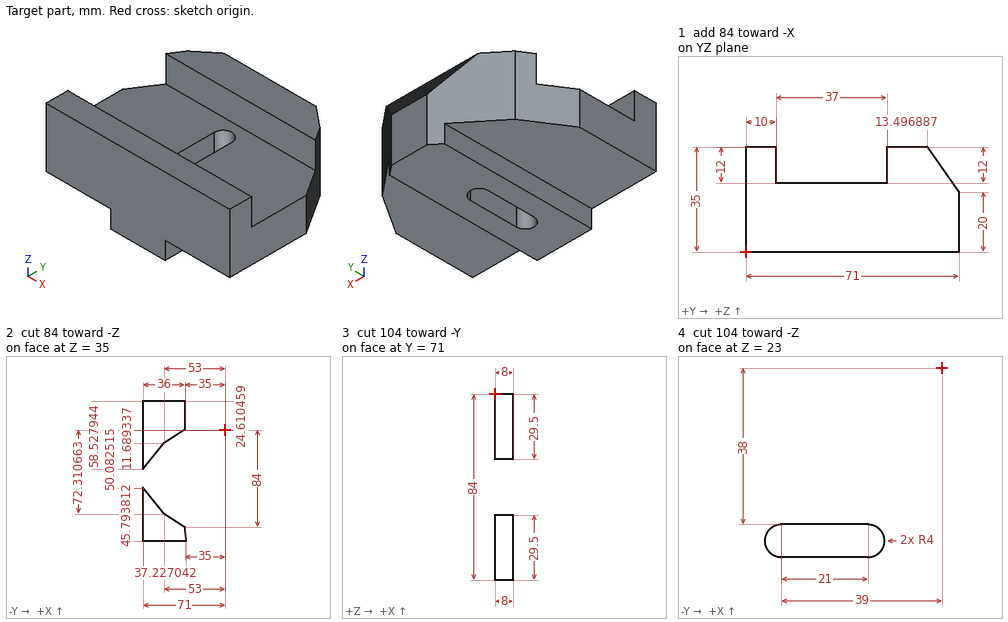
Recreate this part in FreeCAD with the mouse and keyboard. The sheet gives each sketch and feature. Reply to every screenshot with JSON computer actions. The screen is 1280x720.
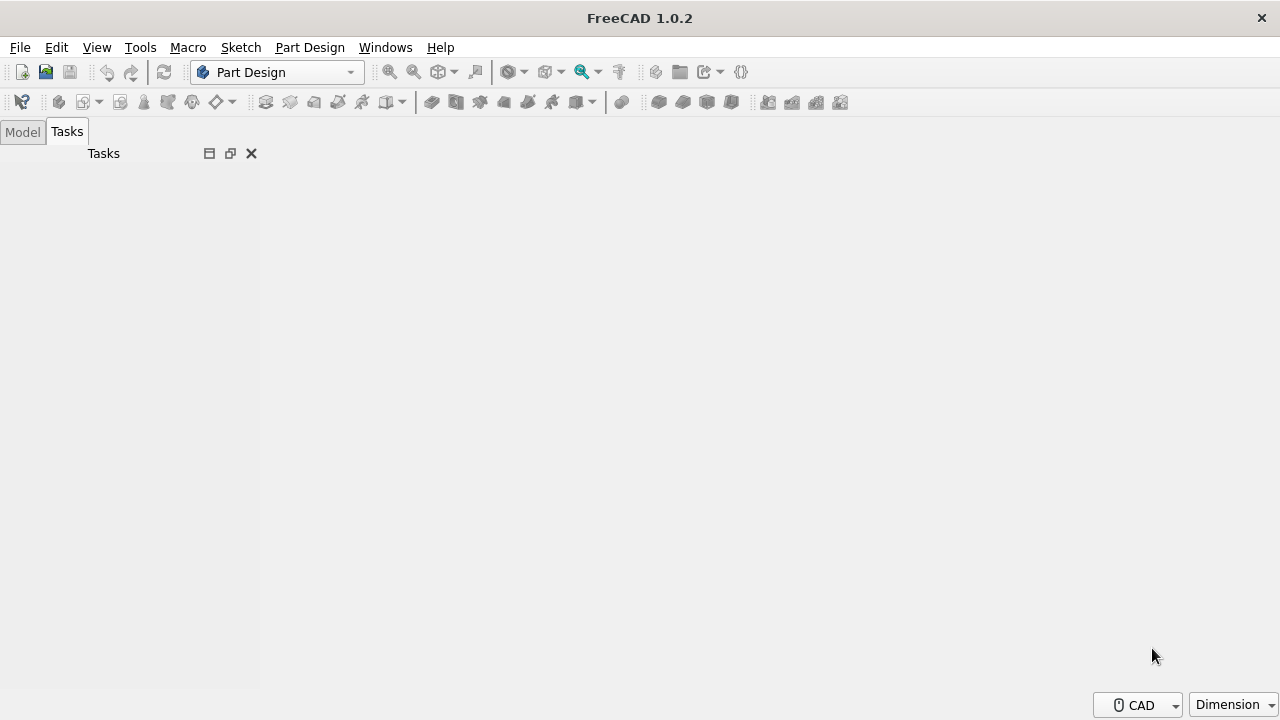
{"action": "left_click", "coordinate": [22, 72]}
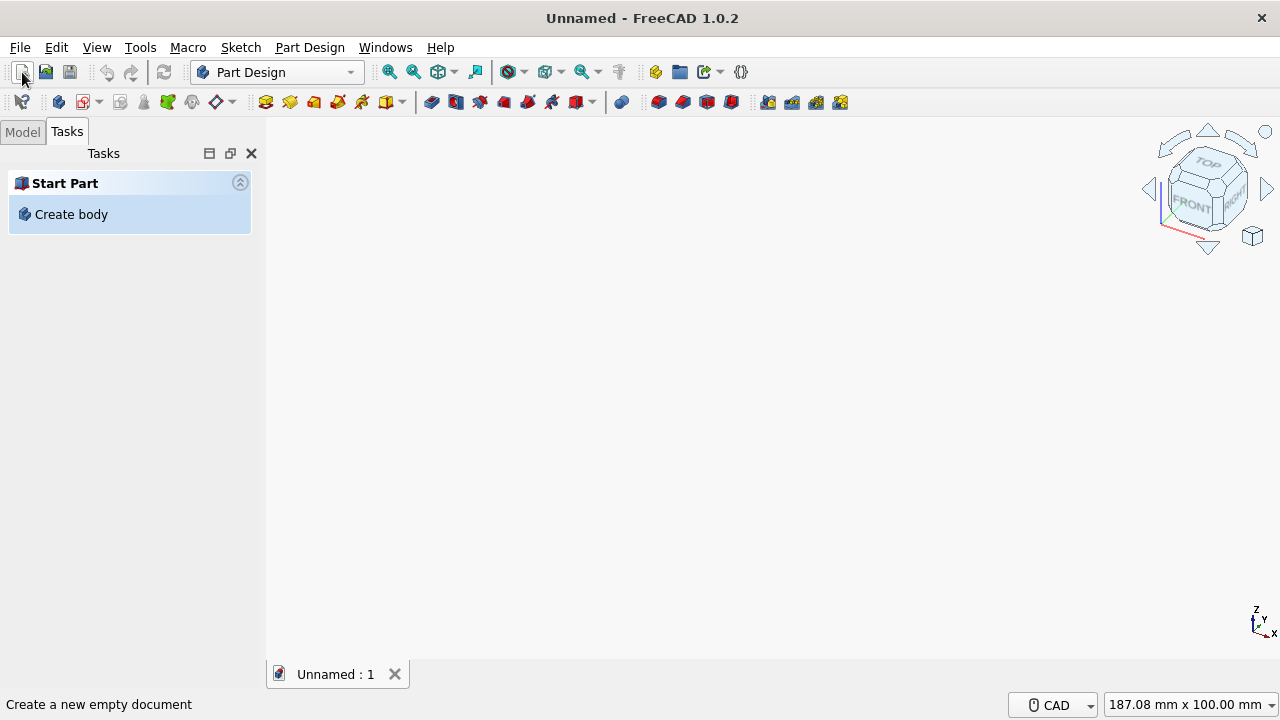
{"action": "left_click", "coordinate": [84, 102]}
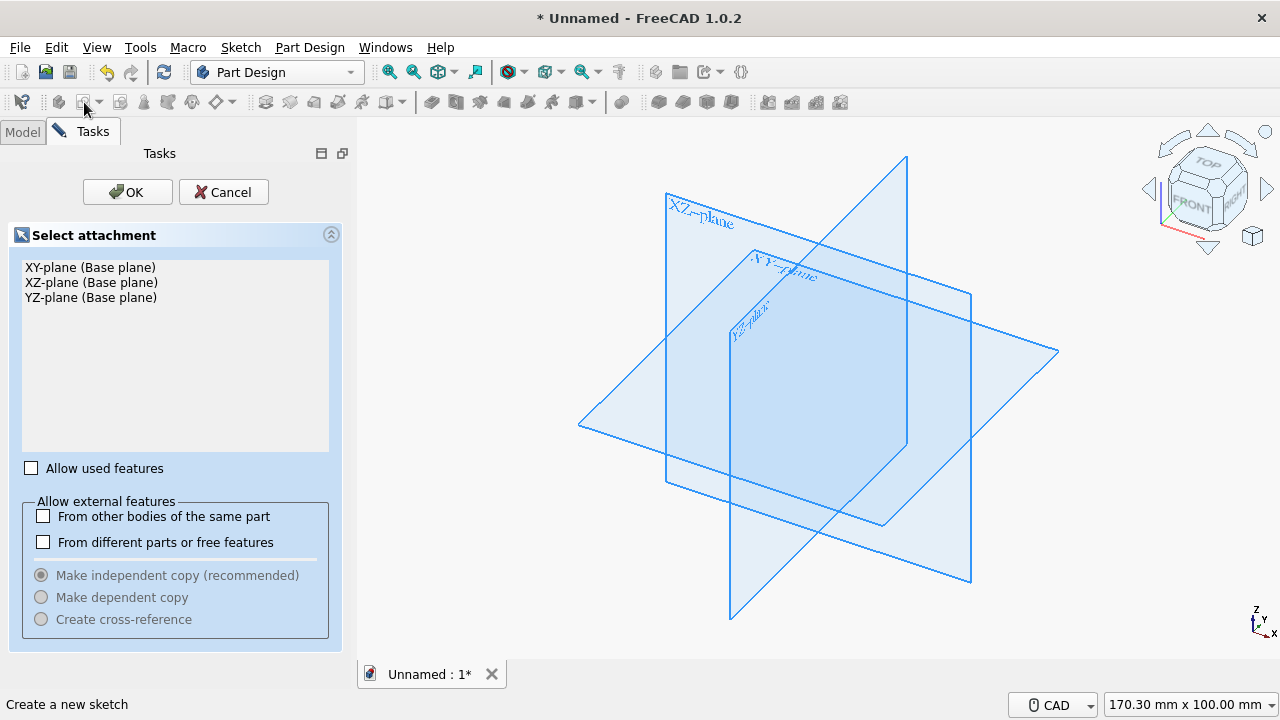
{"action": "left_click", "coordinate": [82, 298]}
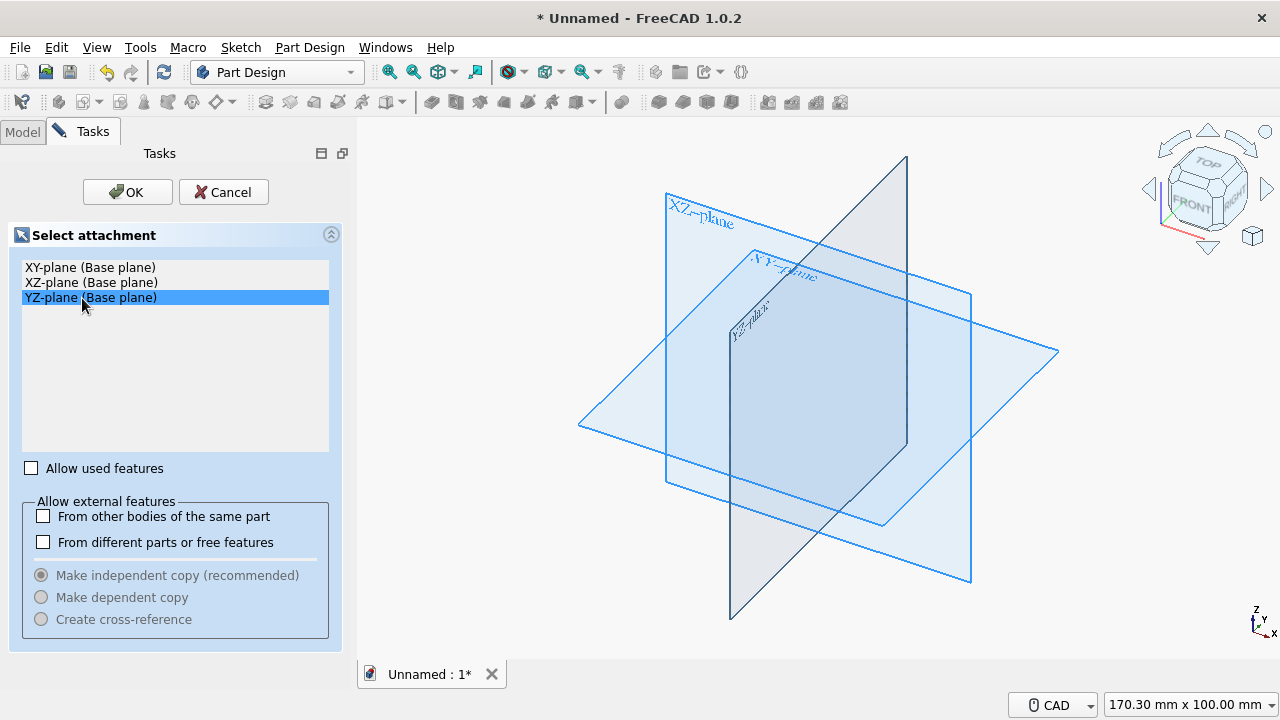
{"action": "left_click", "coordinate": [128, 192]}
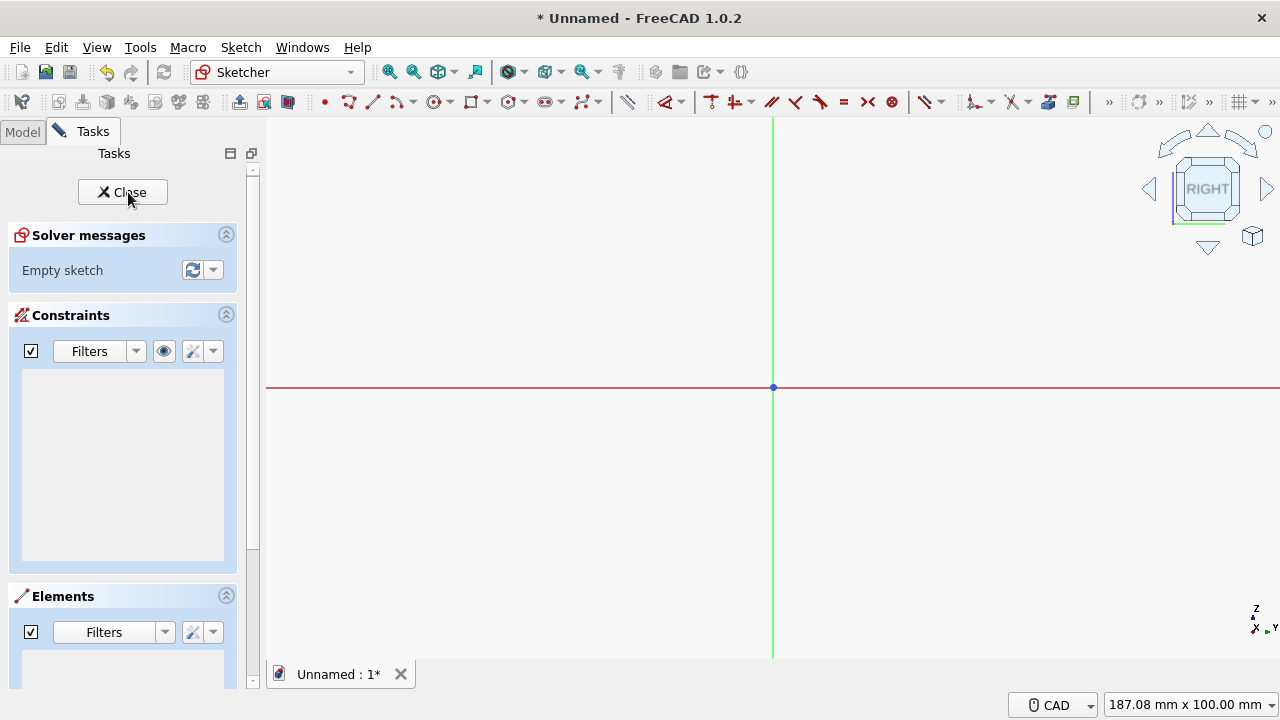
{"action": "scroll", "coordinate": [294, 631], "scroll_direction": "down", "scroll_amount": 1}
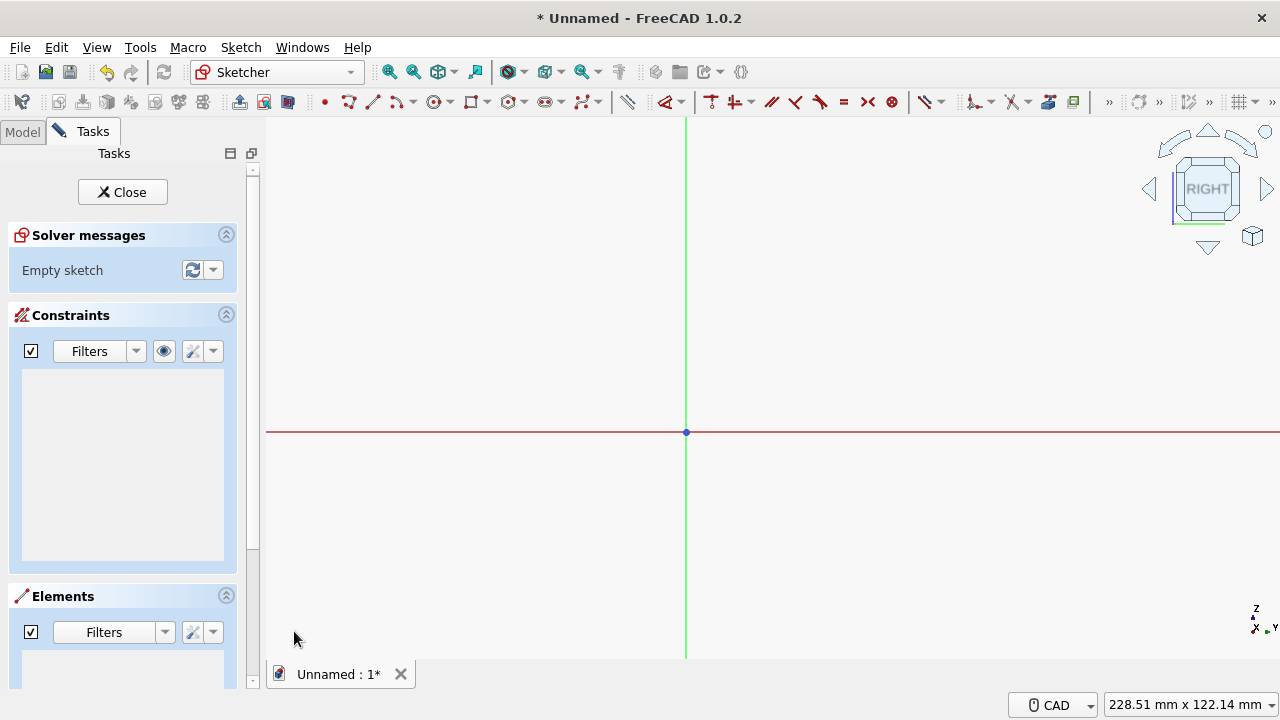
{"action": "scroll", "coordinate": [1013, 314], "scroll_direction": "up", "scroll_amount": 3}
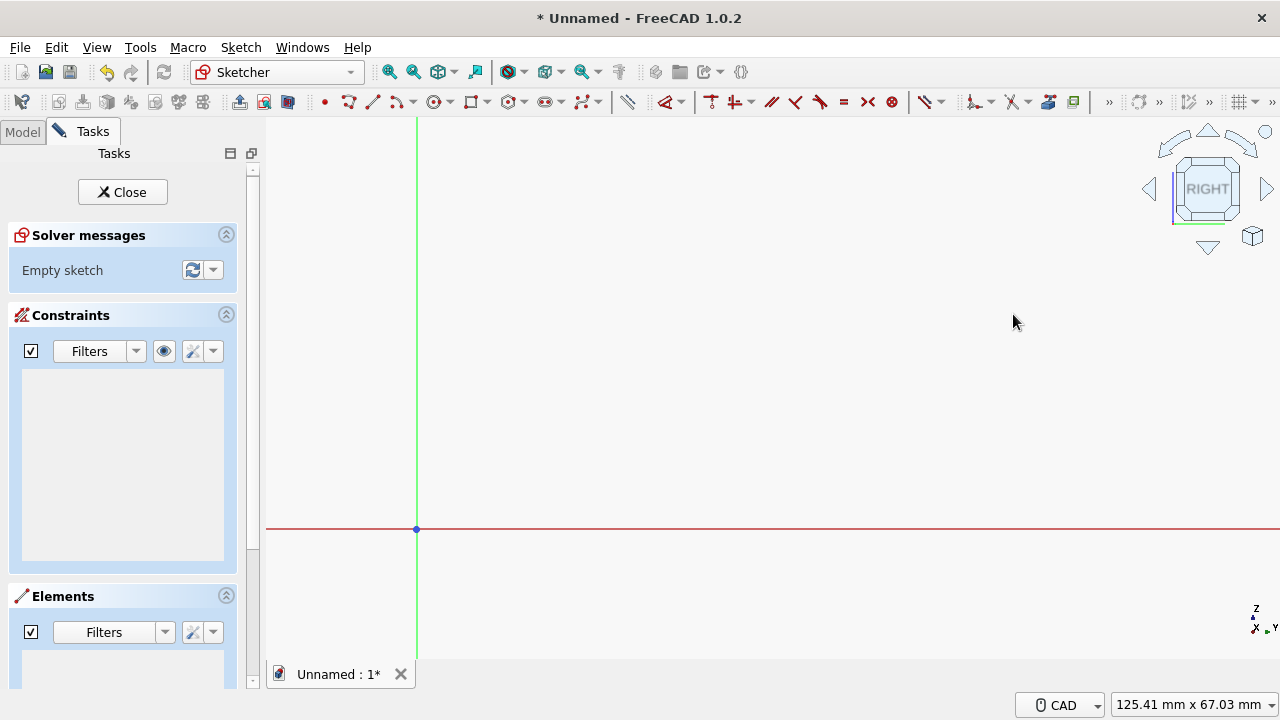
{"action": "left_click", "coordinate": [350, 102]}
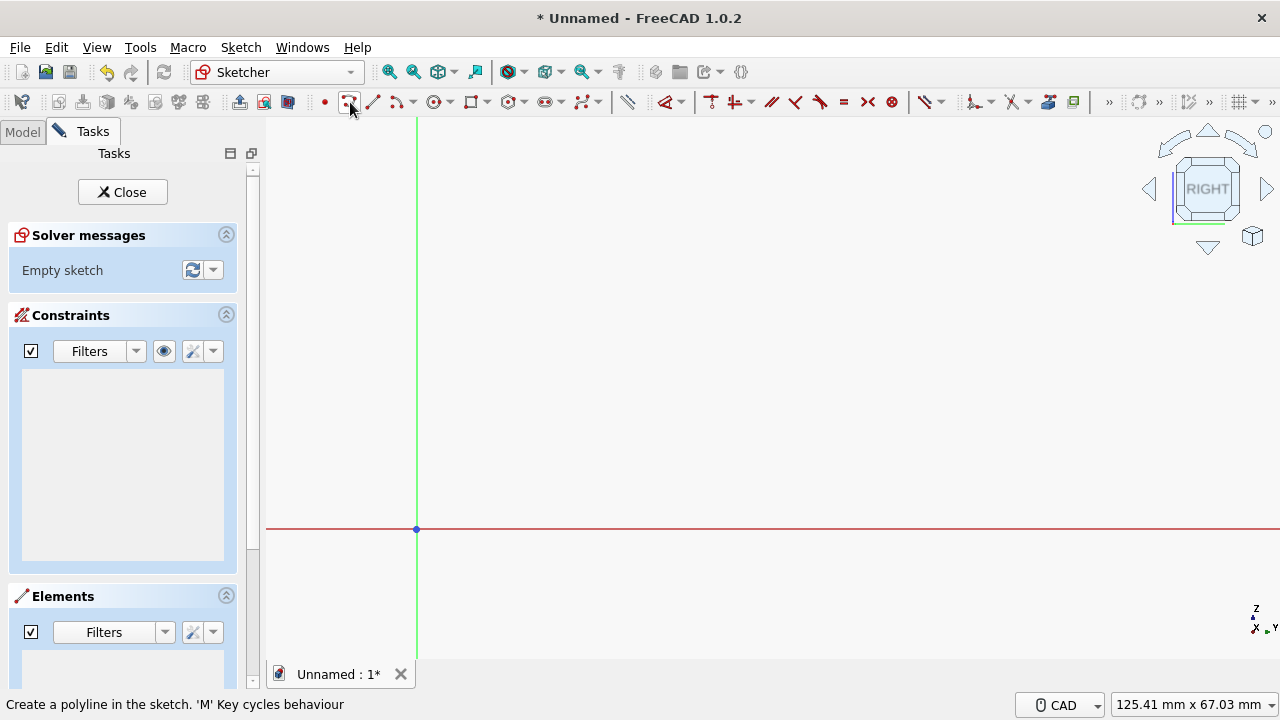
{"action": "left_click", "coordinate": [417, 529]}
{"action": "left_click", "coordinate": [991, 520]}
{"action": "left_click", "coordinate": [991, 367]}
{"action": "left_click", "coordinate": [906, 246]}
{"action": "left_click", "coordinate": [797, 246]}
{"action": "left_click", "coordinate": [797, 343]}
{"action": "left_click", "coordinate": [498, 343]}
{"action": "left_click", "coordinate": [498, 246]}
{"action": "left_click", "coordinate": [426, 246]}
{"action": "left_click", "coordinate": [417, 529]}
{"action": "key", "text": "Escape"}
{"action": "key", "text": "Escape"}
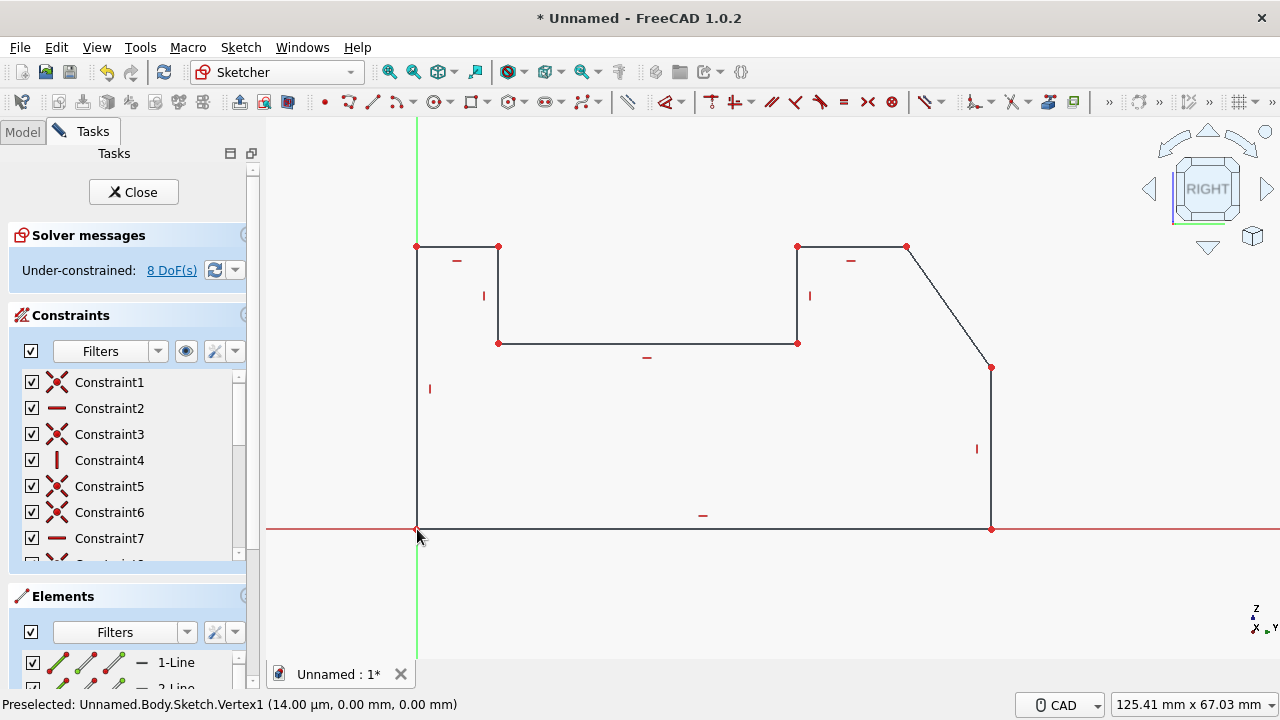
{"action": "left_click", "coordinate": [589, 529]}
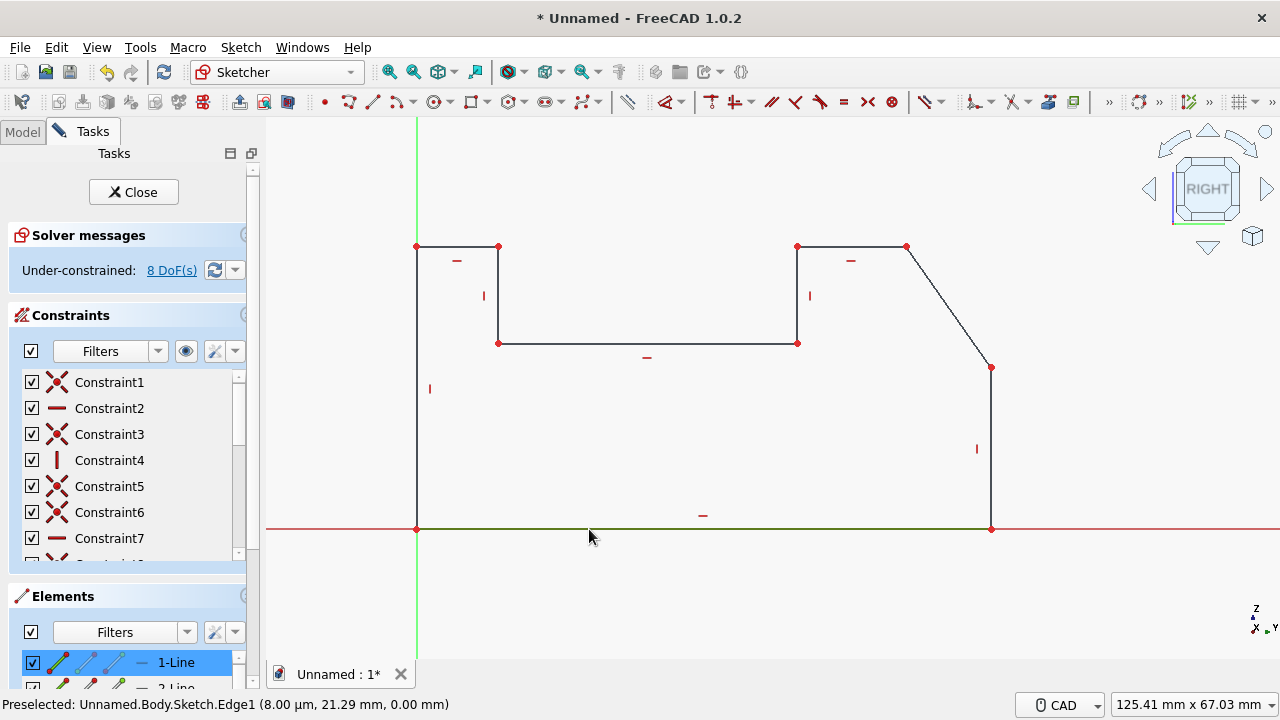
{"action": "left_click", "coordinate": [684, 102]}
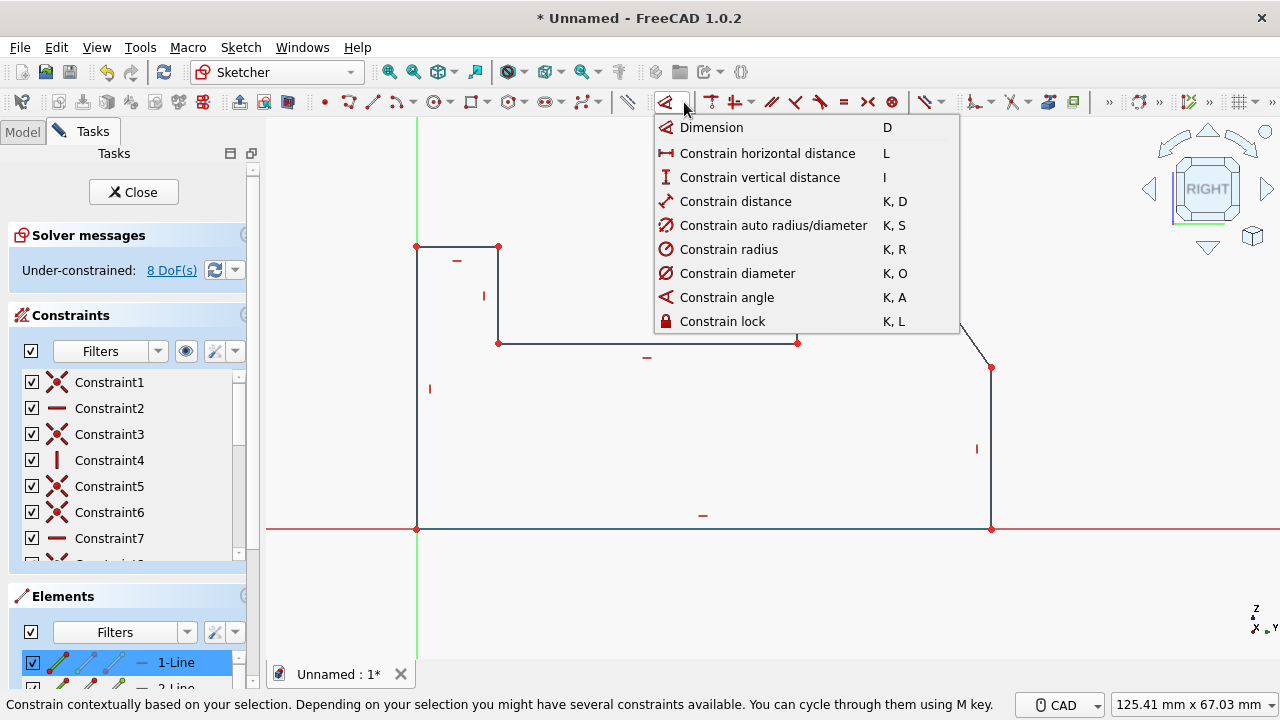
{"action": "left_click", "coordinate": [807, 153]}